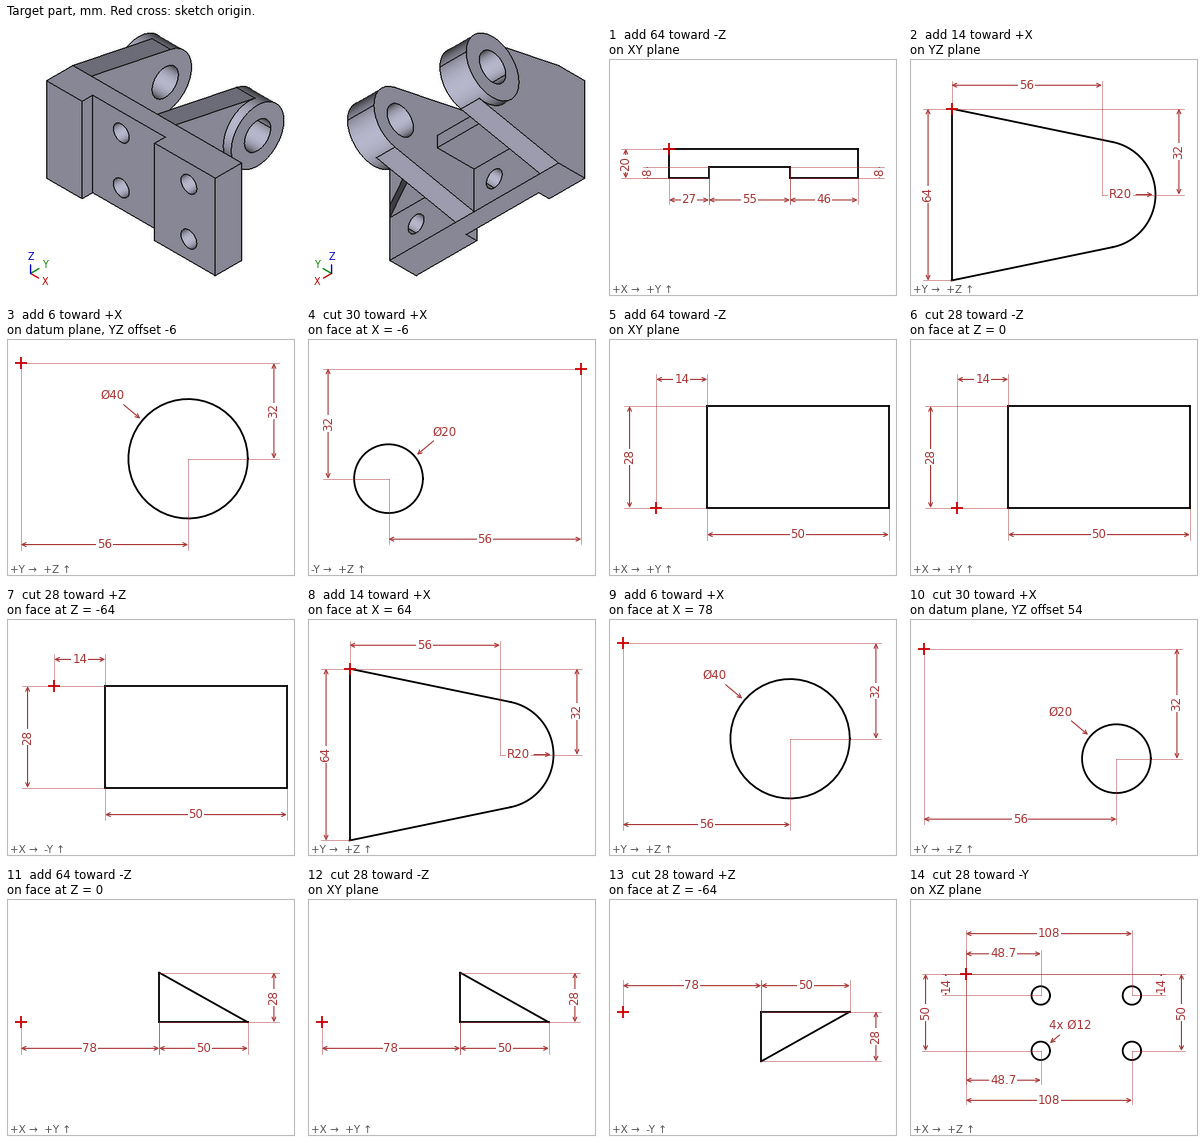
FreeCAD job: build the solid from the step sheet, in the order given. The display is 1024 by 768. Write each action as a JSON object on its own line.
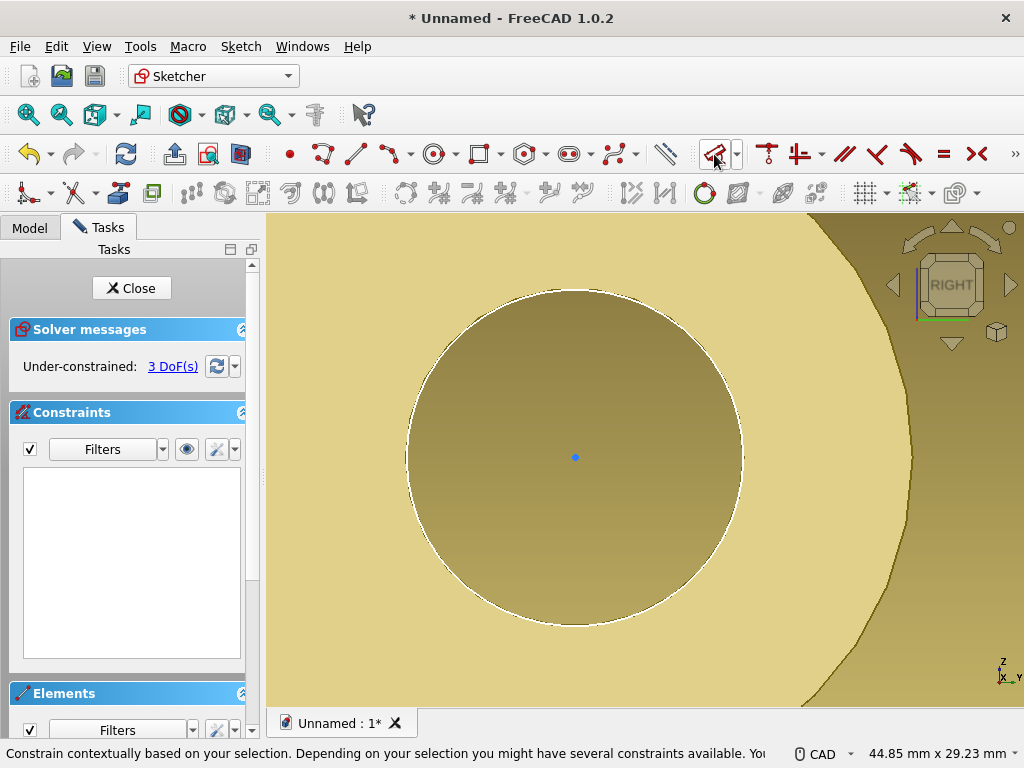
{"action": "left_click", "coordinate": [694, 339]}
{"action": "left_click", "coordinate": [717, 316]}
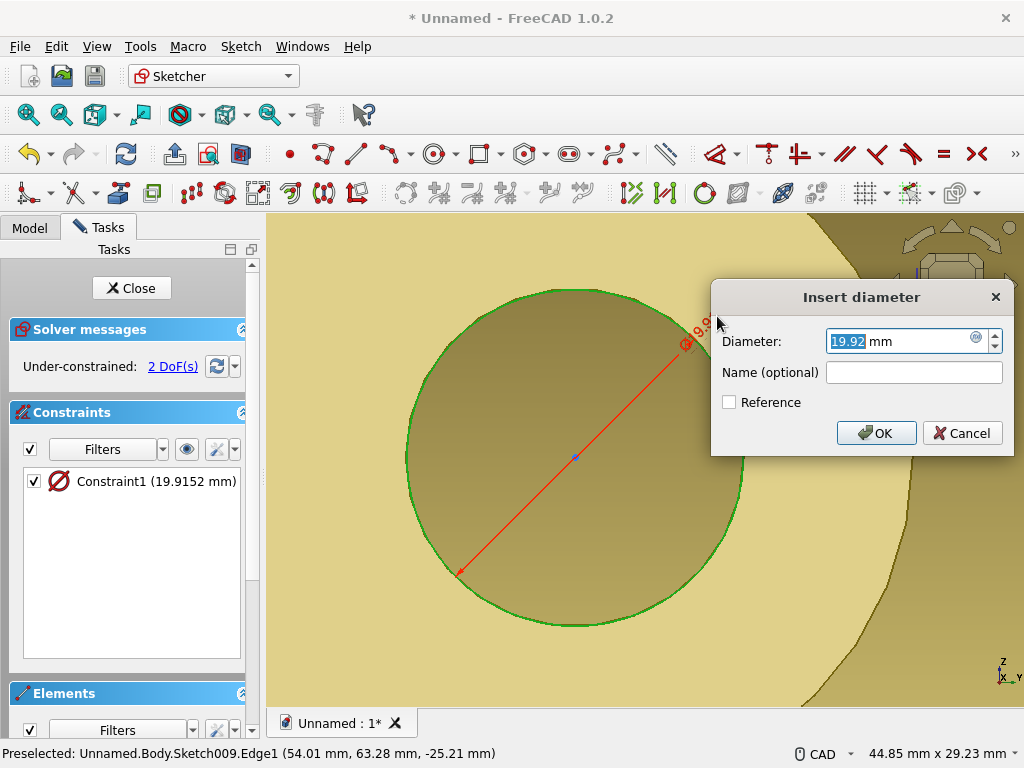
{"action": "type", "text": "20"}
{"action": "key", "text": "Return"}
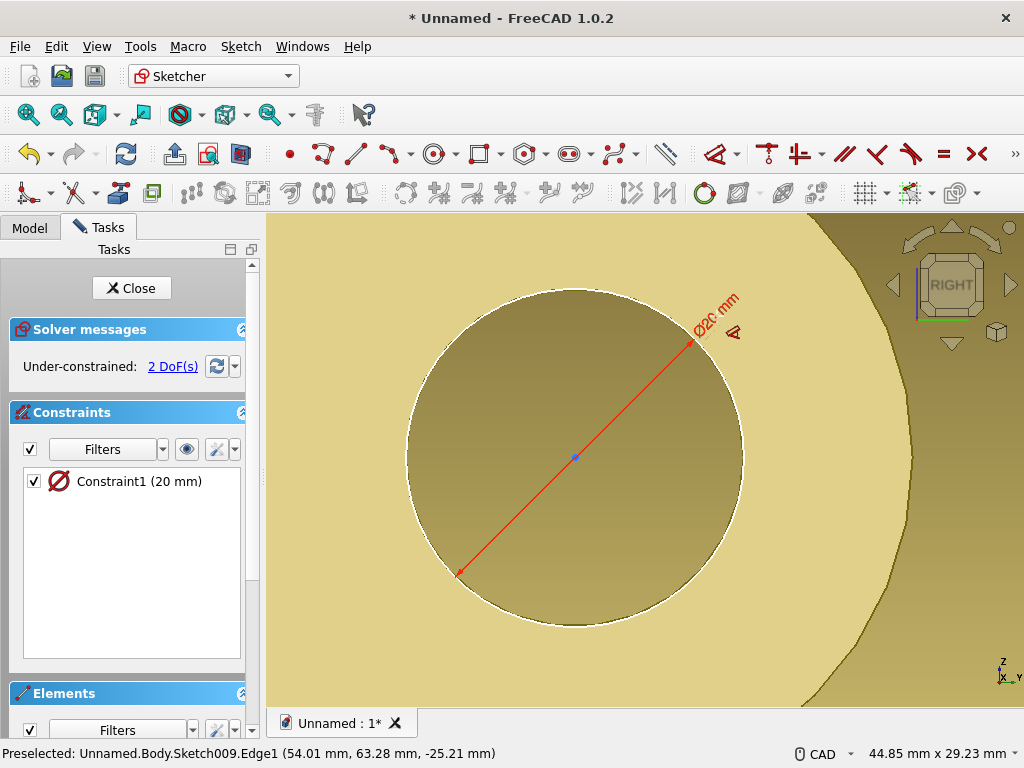
{"action": "left_click", "coordinate": [575, 458]}
{"action": "left_click", "coordinate": [435, 492]}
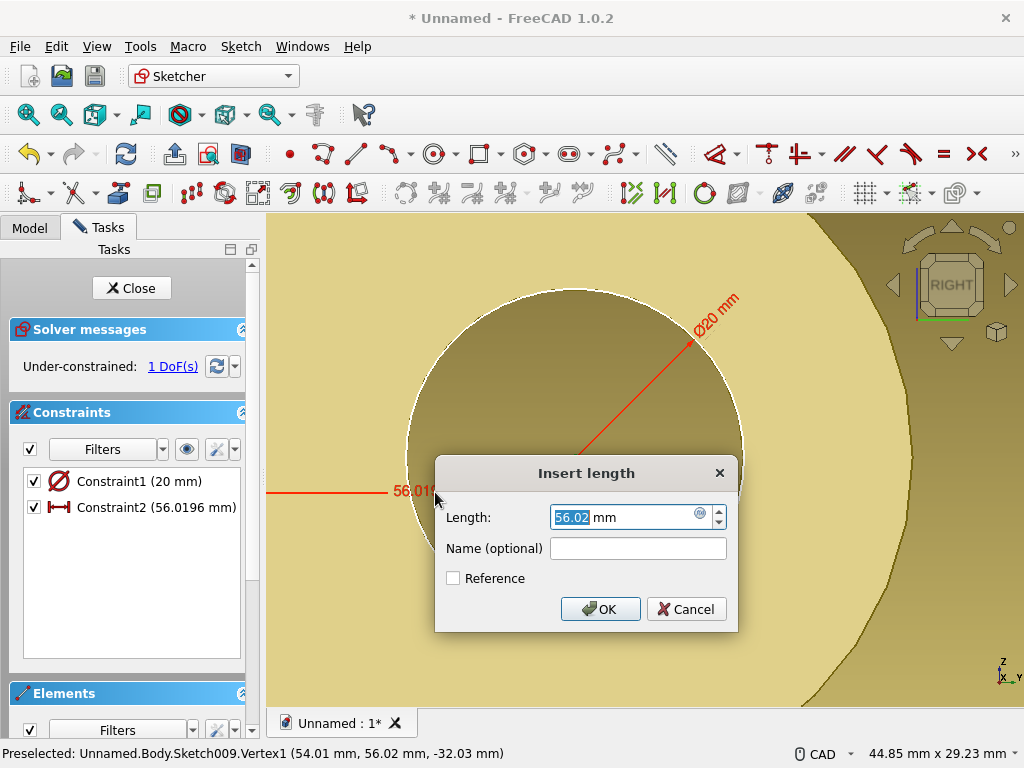
{"action": "type", "text": "56"}
{"action": "key", "text": "Return"}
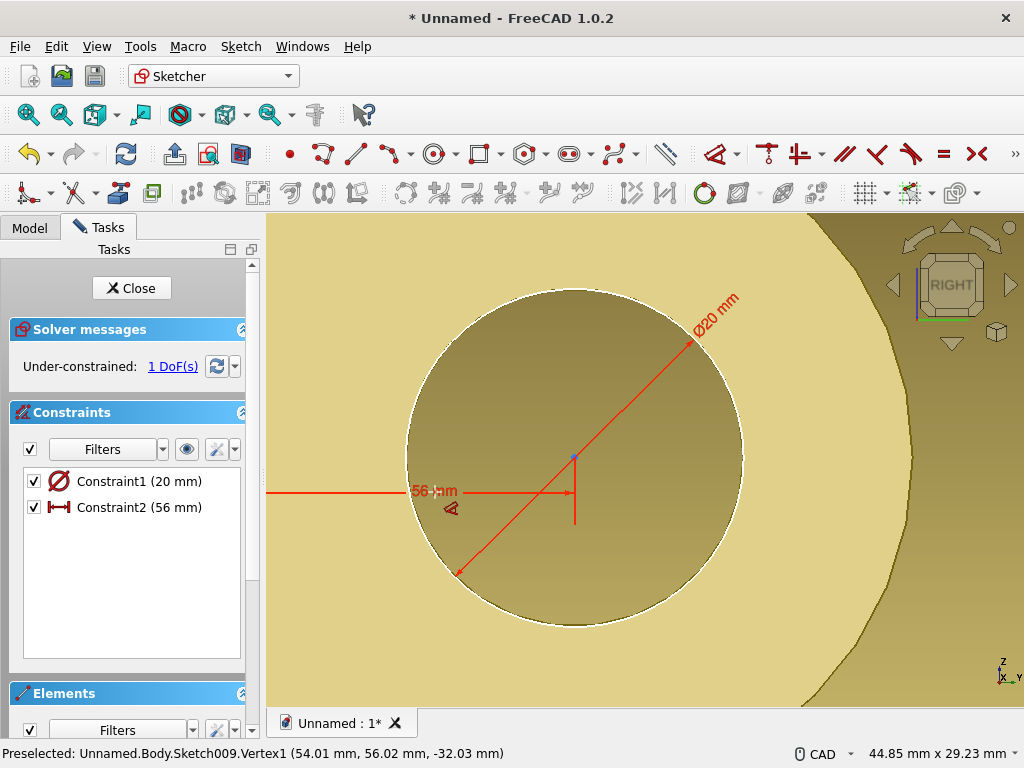
{"action": "left_click", "coordinate": [575, 458]}
{"action": "left_click", "coordinate": [609, 349]}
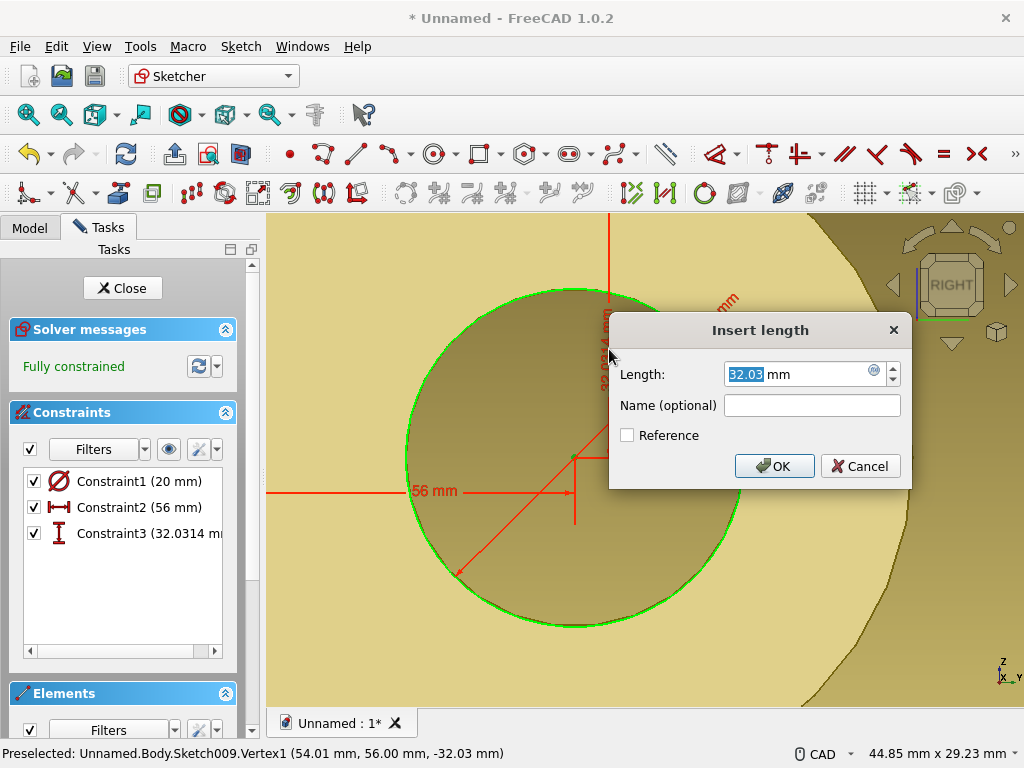
{"action": "type", "text": "32"}
{"action": "key", "text": "Return"}
{"action": "key", "text": "Escape"}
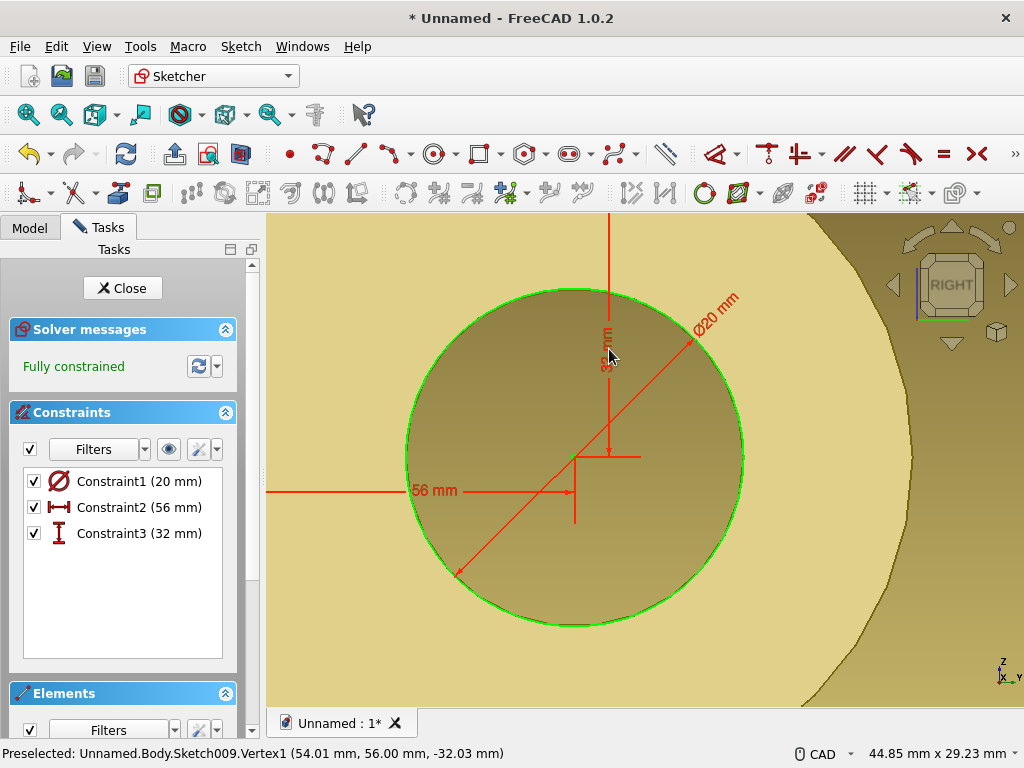
{"action": "left_click", "coordinate": [123, 288]}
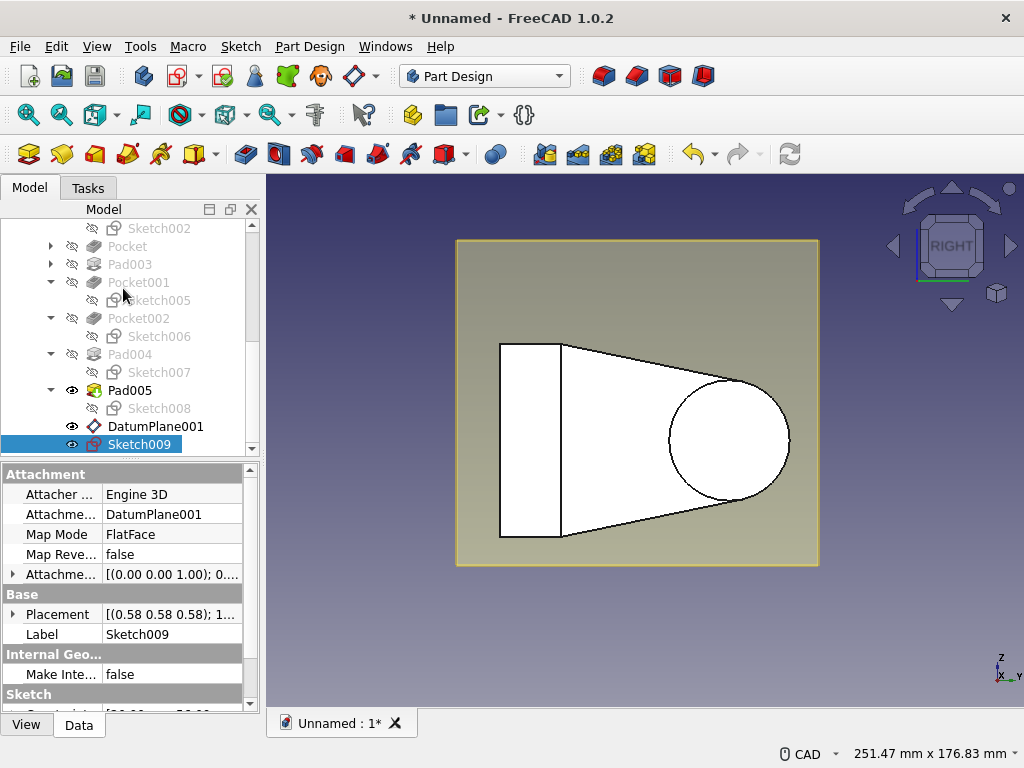
{"action": "left_click", "coordinate": [246, 154]}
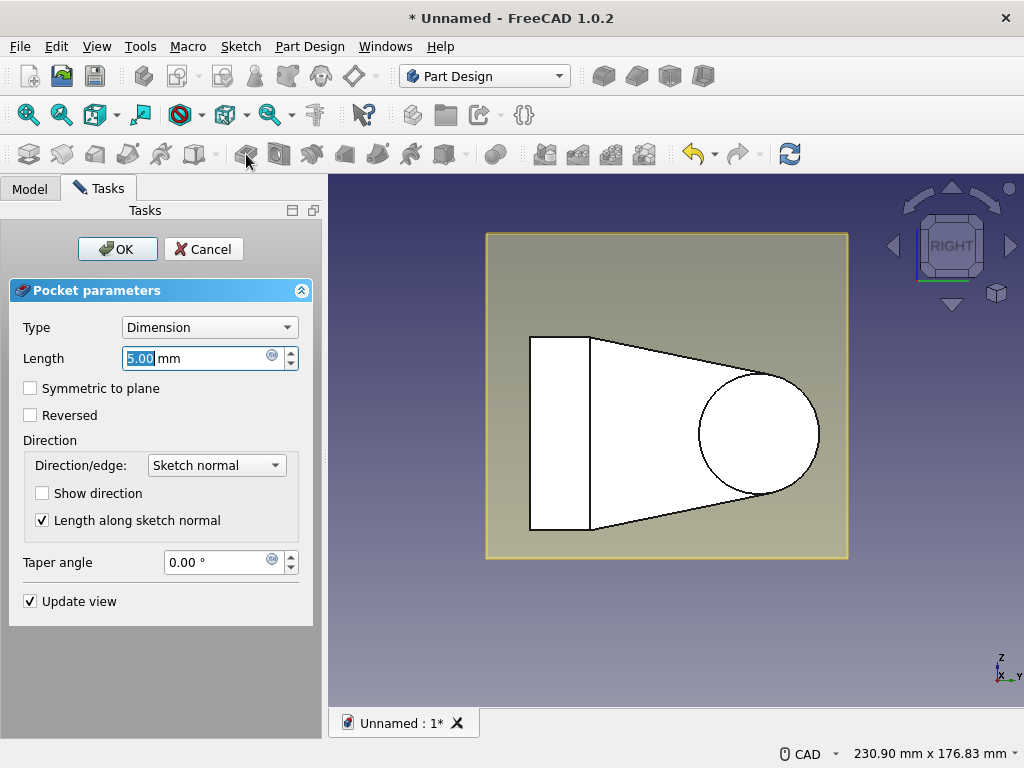
{"action": "type", "text": "30"}
{"action": "key", "text": "Tab"}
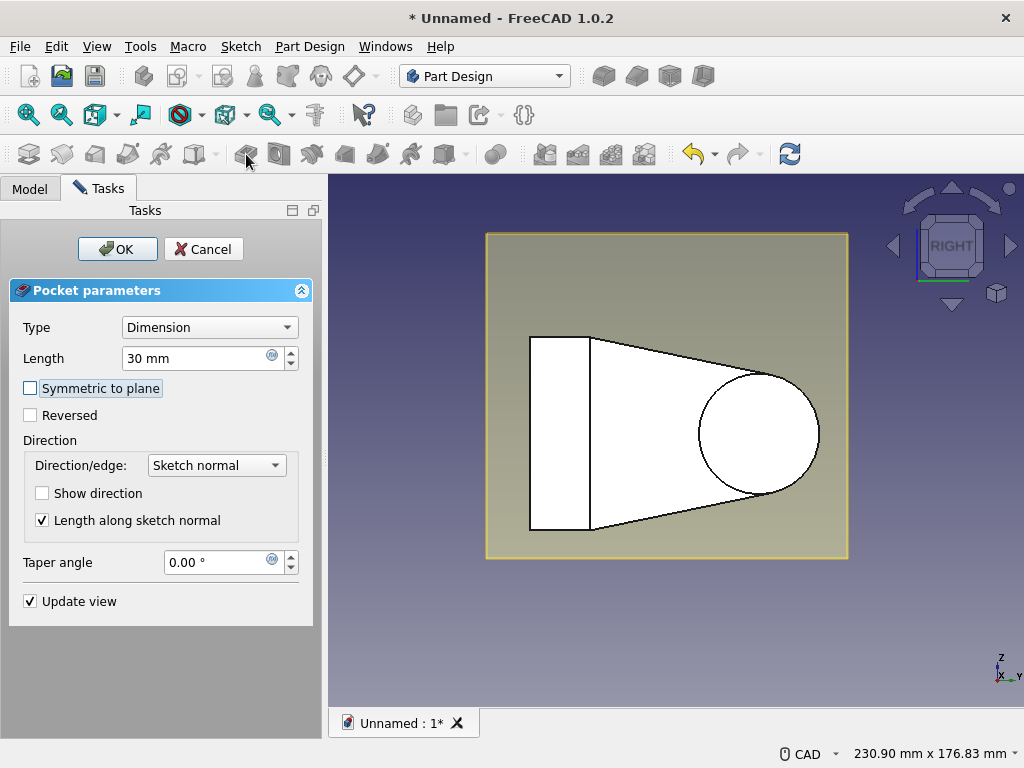
{"action": "left_click", "coordinate": [31, 415]}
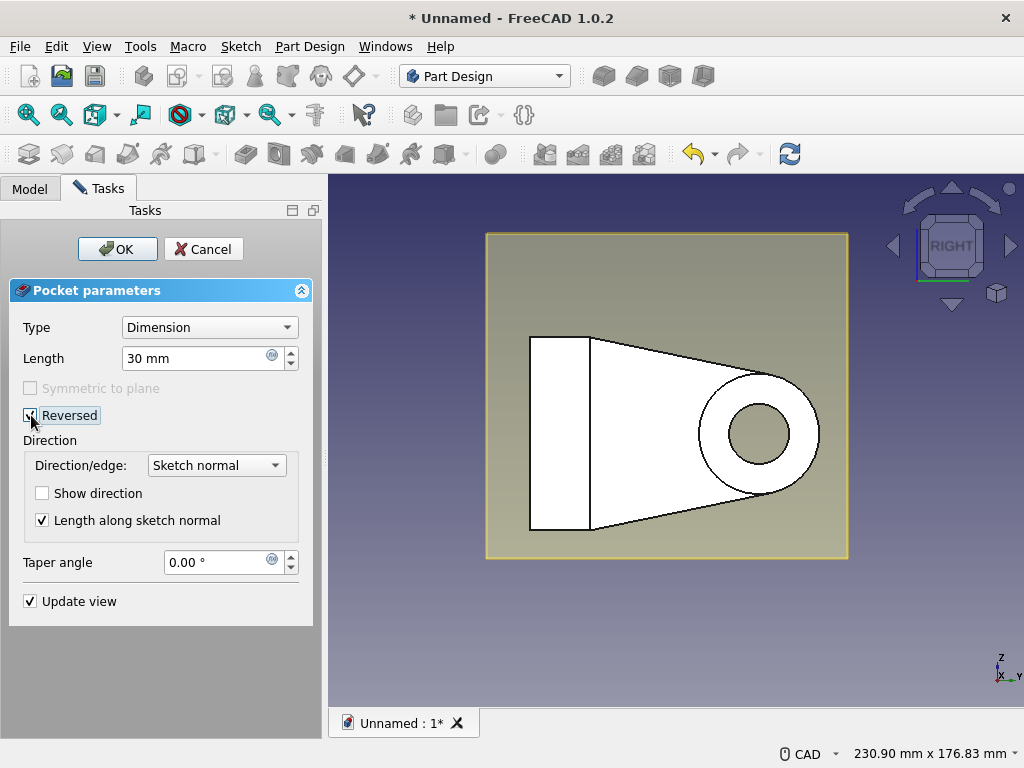
{"action": "left_click", "coordinate": [118, 249]}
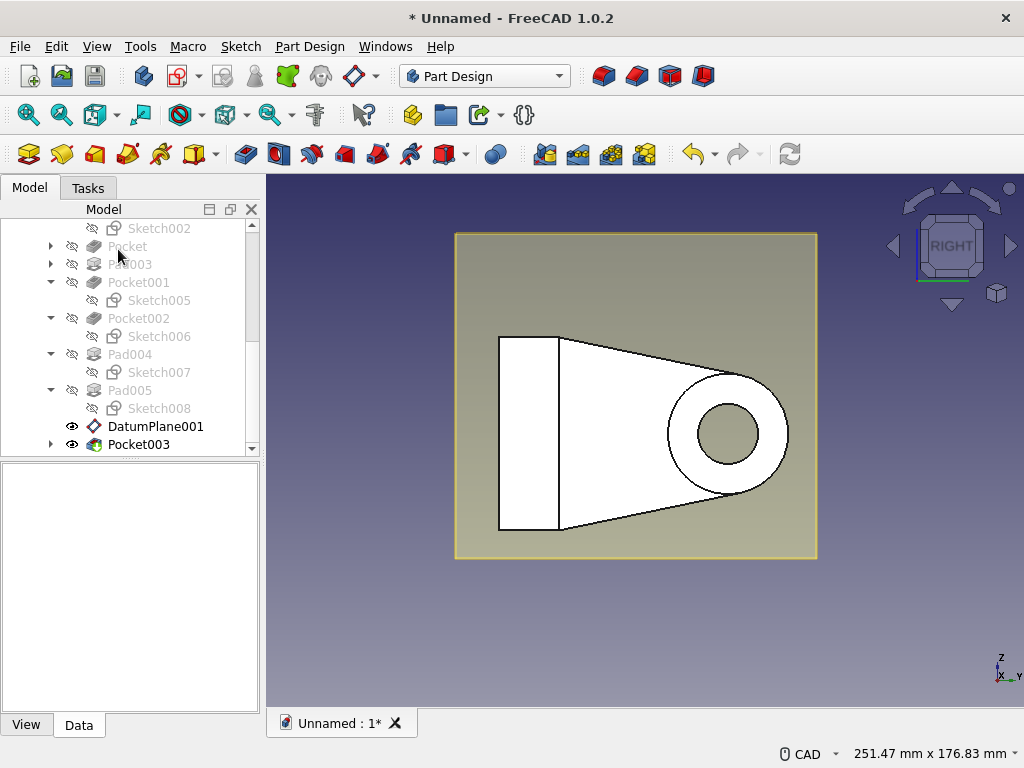
{"action": "left_click", "coordinate": [117, 426]}
{"action": "key", "text": "space"}